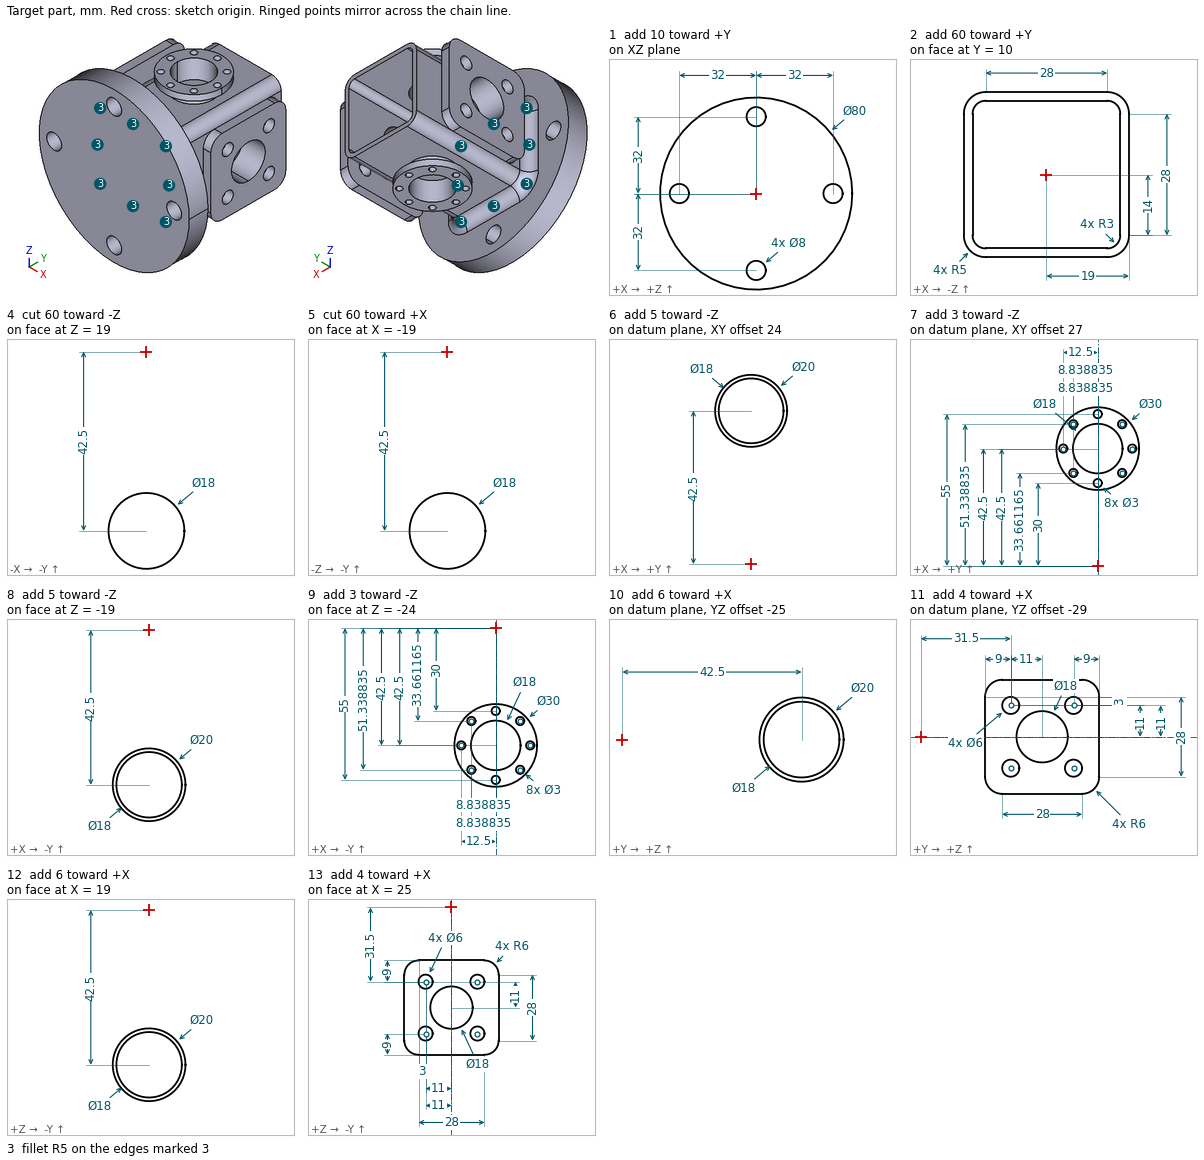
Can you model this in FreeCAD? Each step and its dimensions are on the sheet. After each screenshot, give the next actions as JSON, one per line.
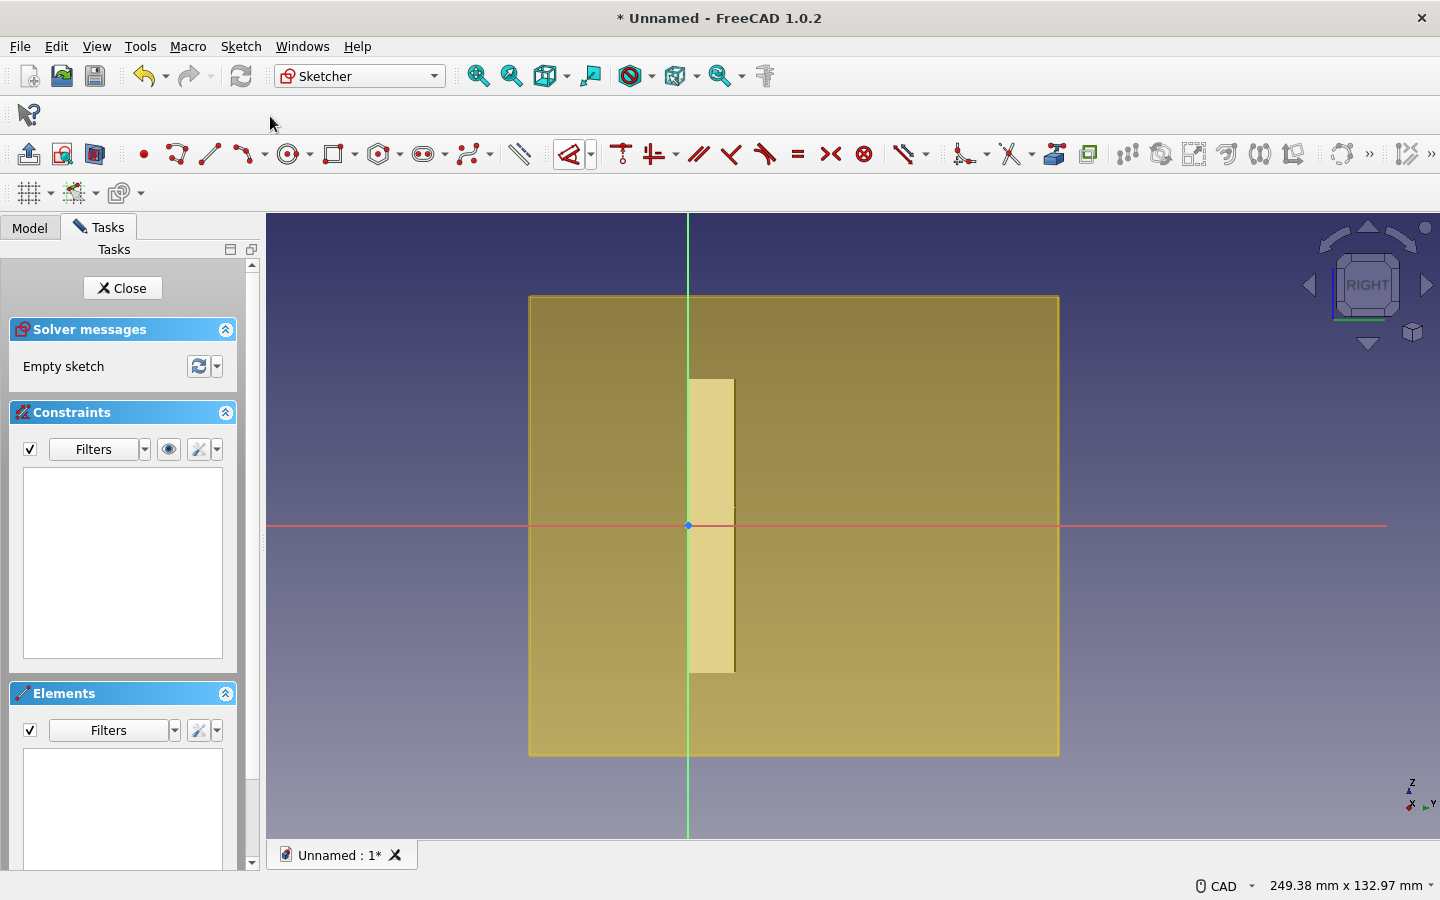
{"action": "scroll", "coordinate": [922, 526], "scroll_direction": "up", "scroll_amount": 7}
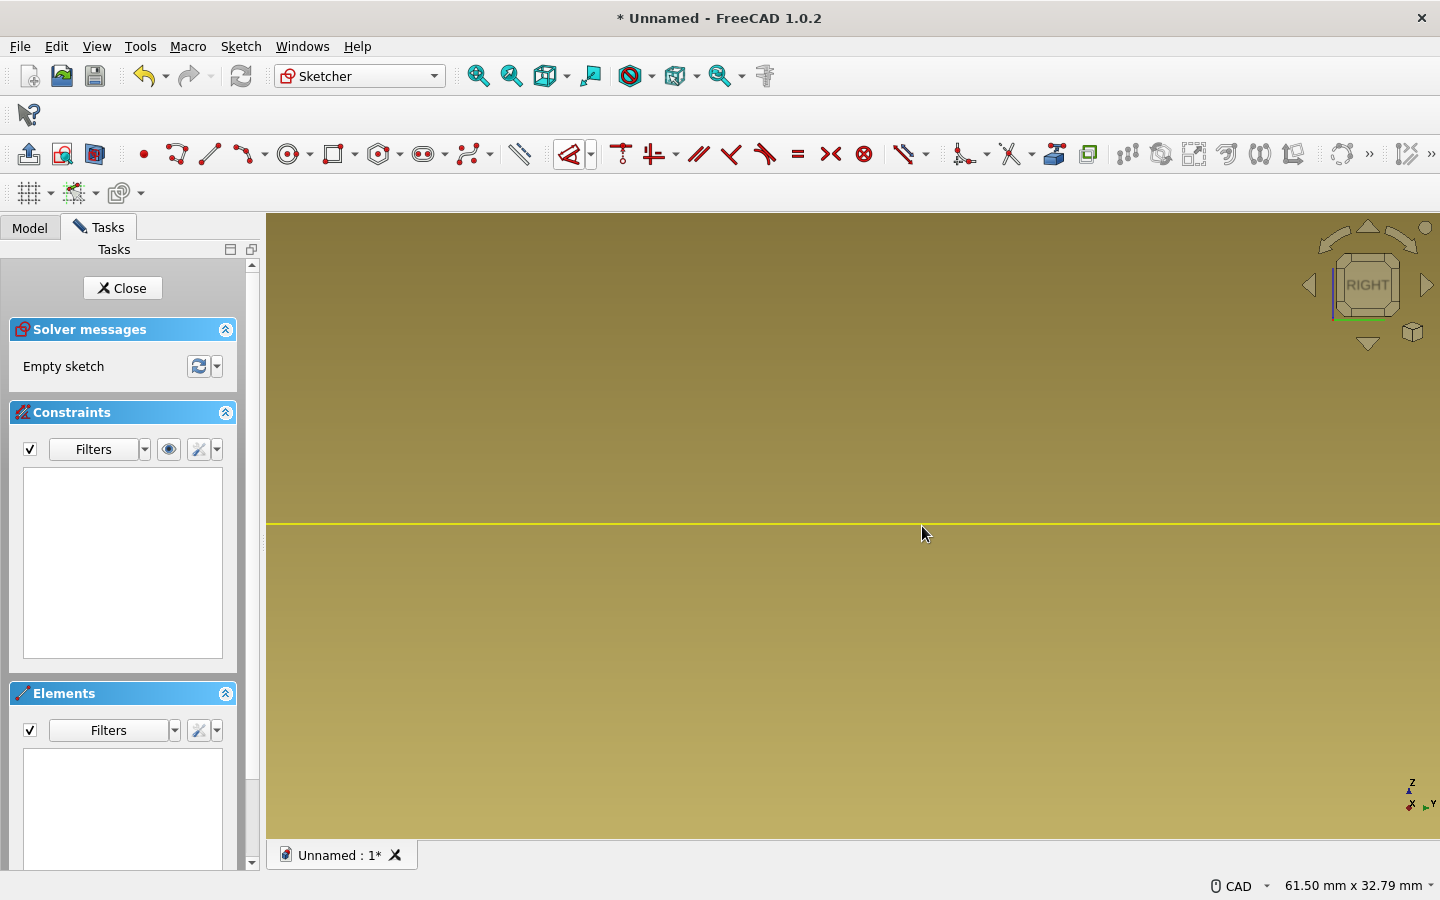
{"action": "key", "text": "g c"}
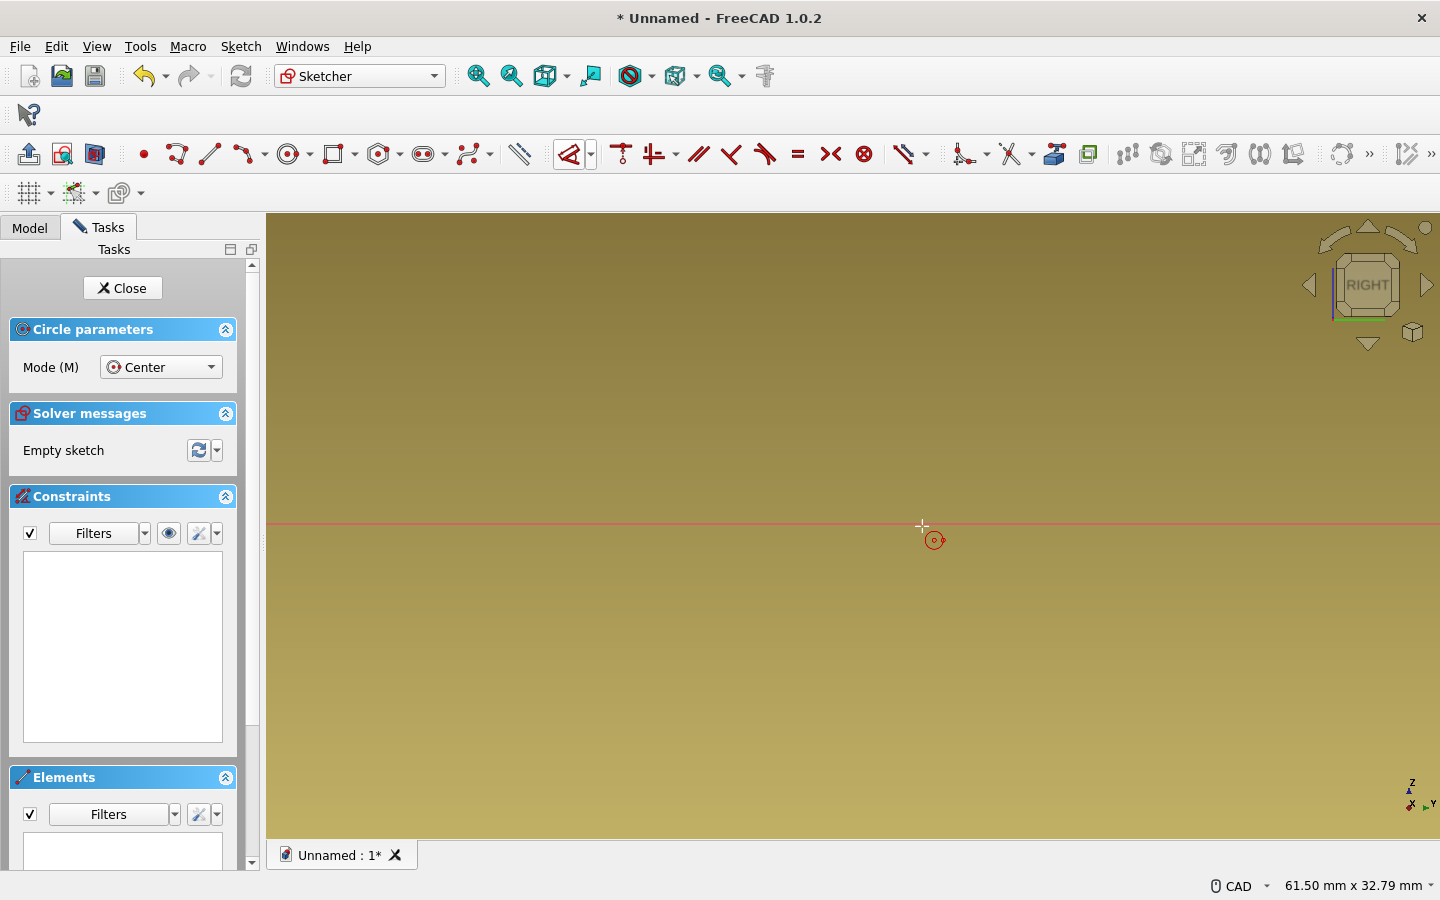
{"action": "left_click", "coordinate": [784, 524]}
{"action": "mouse_move", "coordinate": [919, 389]}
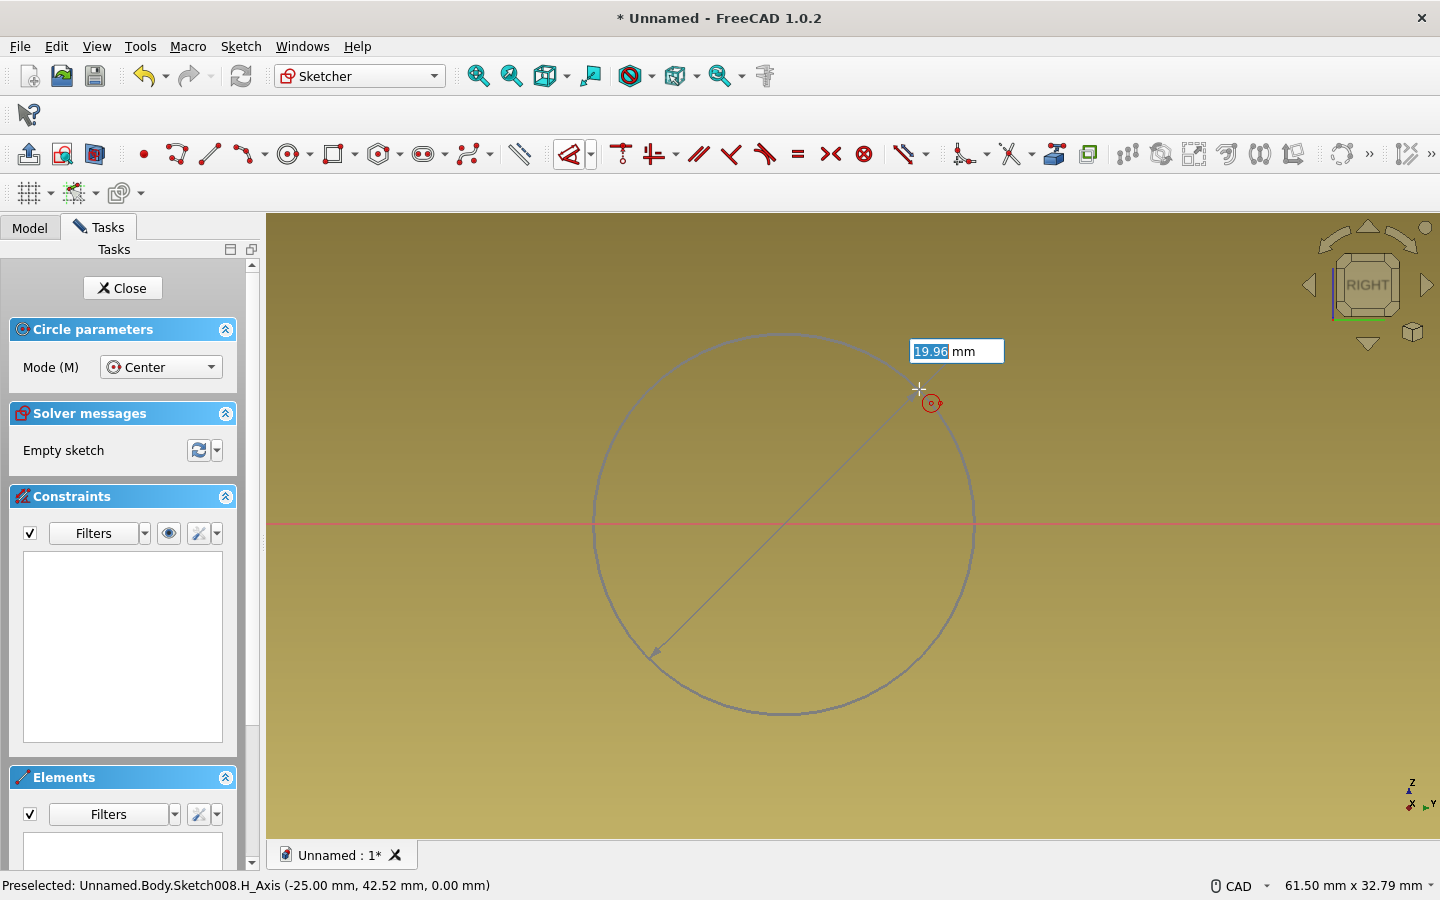
{"action": "type", "text": "20"}
{"action": "key", "text": "Return"}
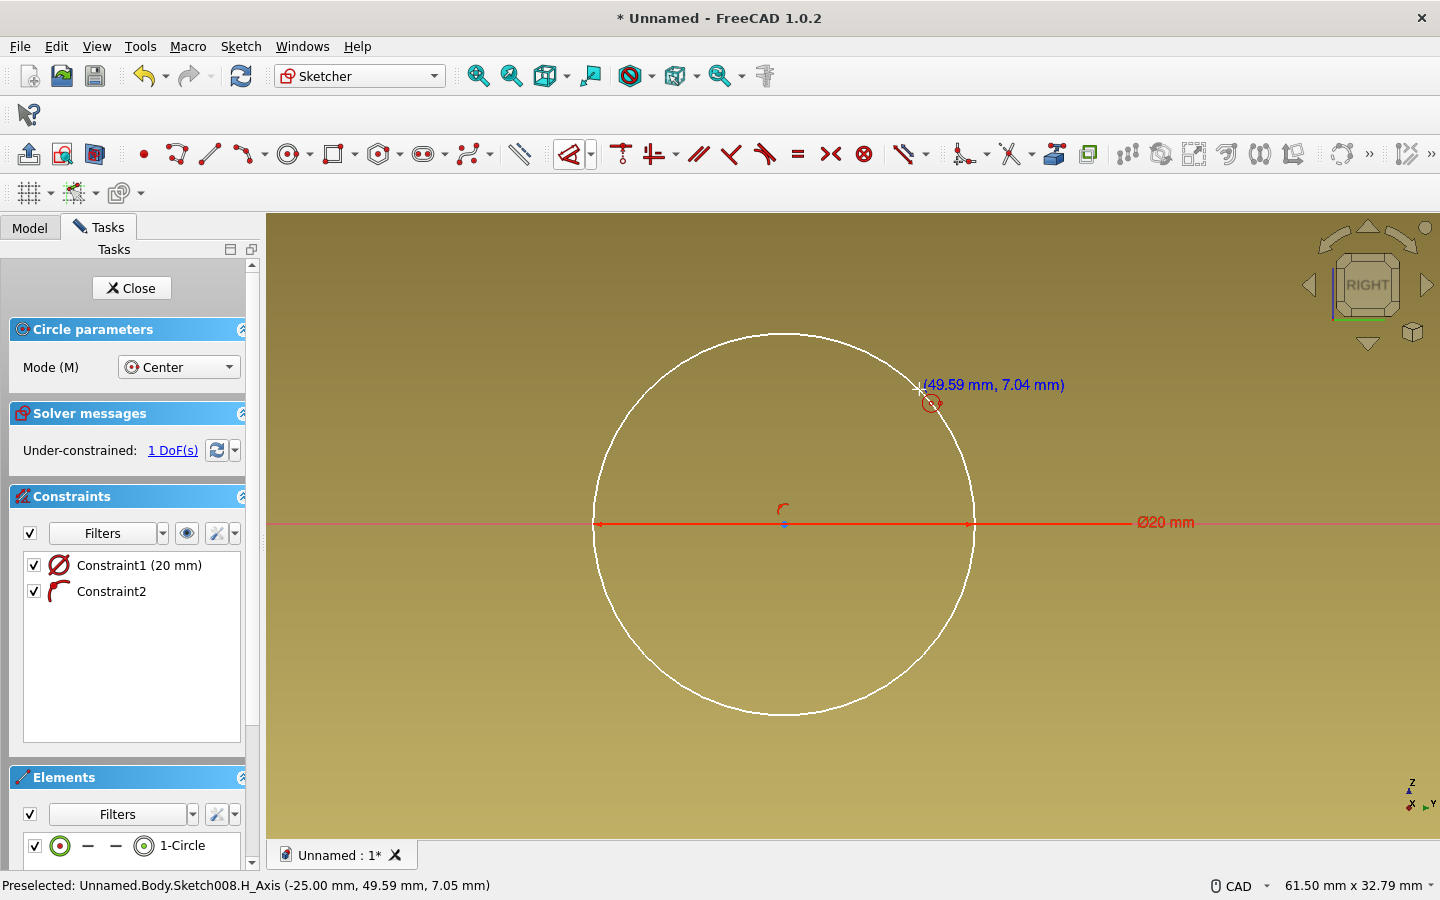
{"action": "left_click", "coordinate": [784, 524]}
{"action": "mouse_move", "coordinate": [905, 403]}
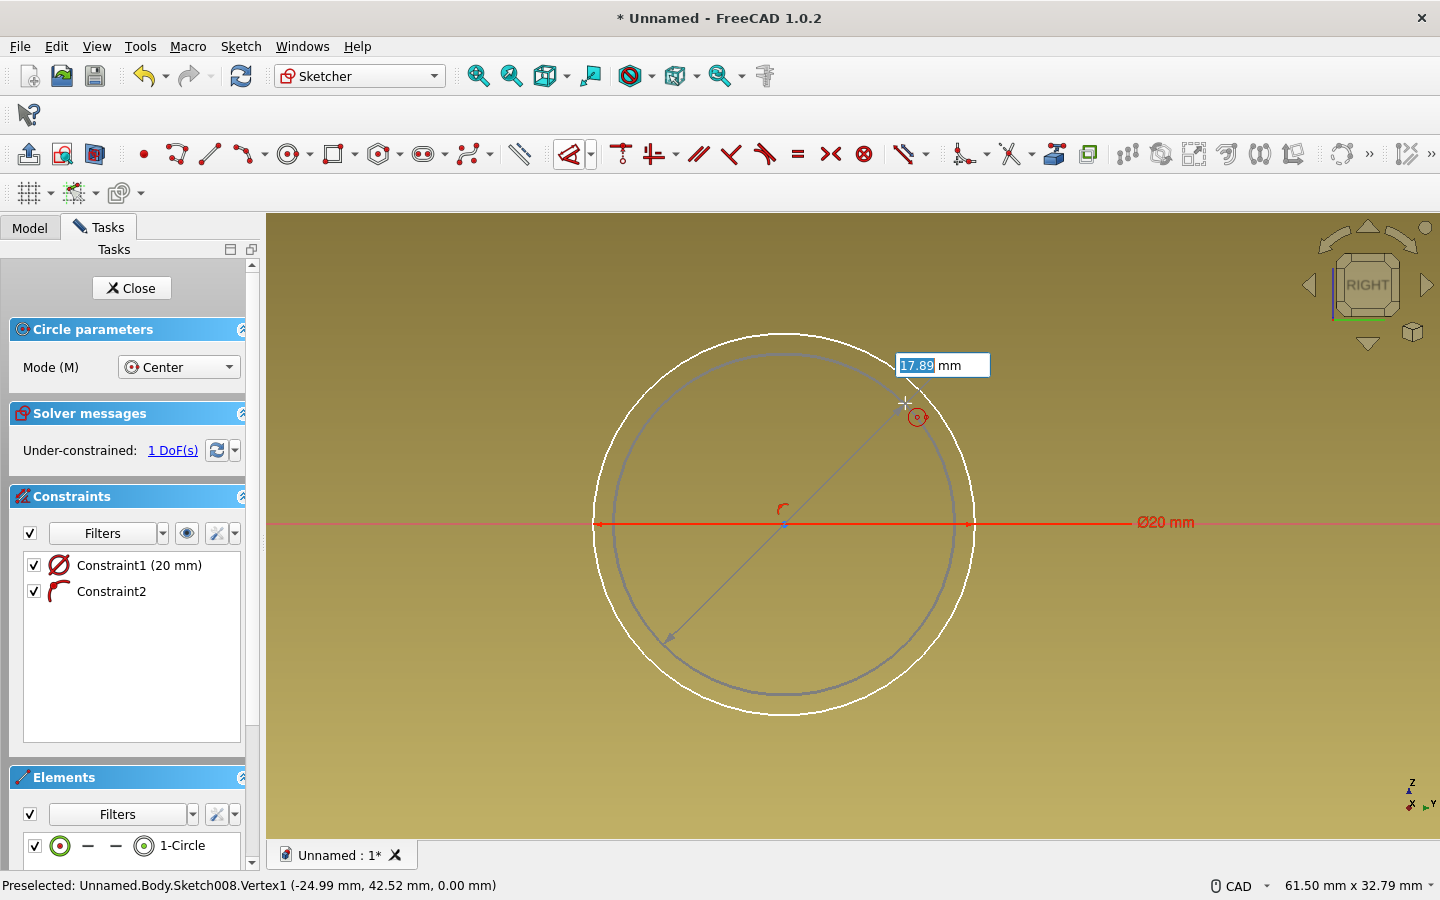
{"action": "type", "text": "18"}
{"action": "key", "text": "Return"}
{"action": "key", "text": "Escape"}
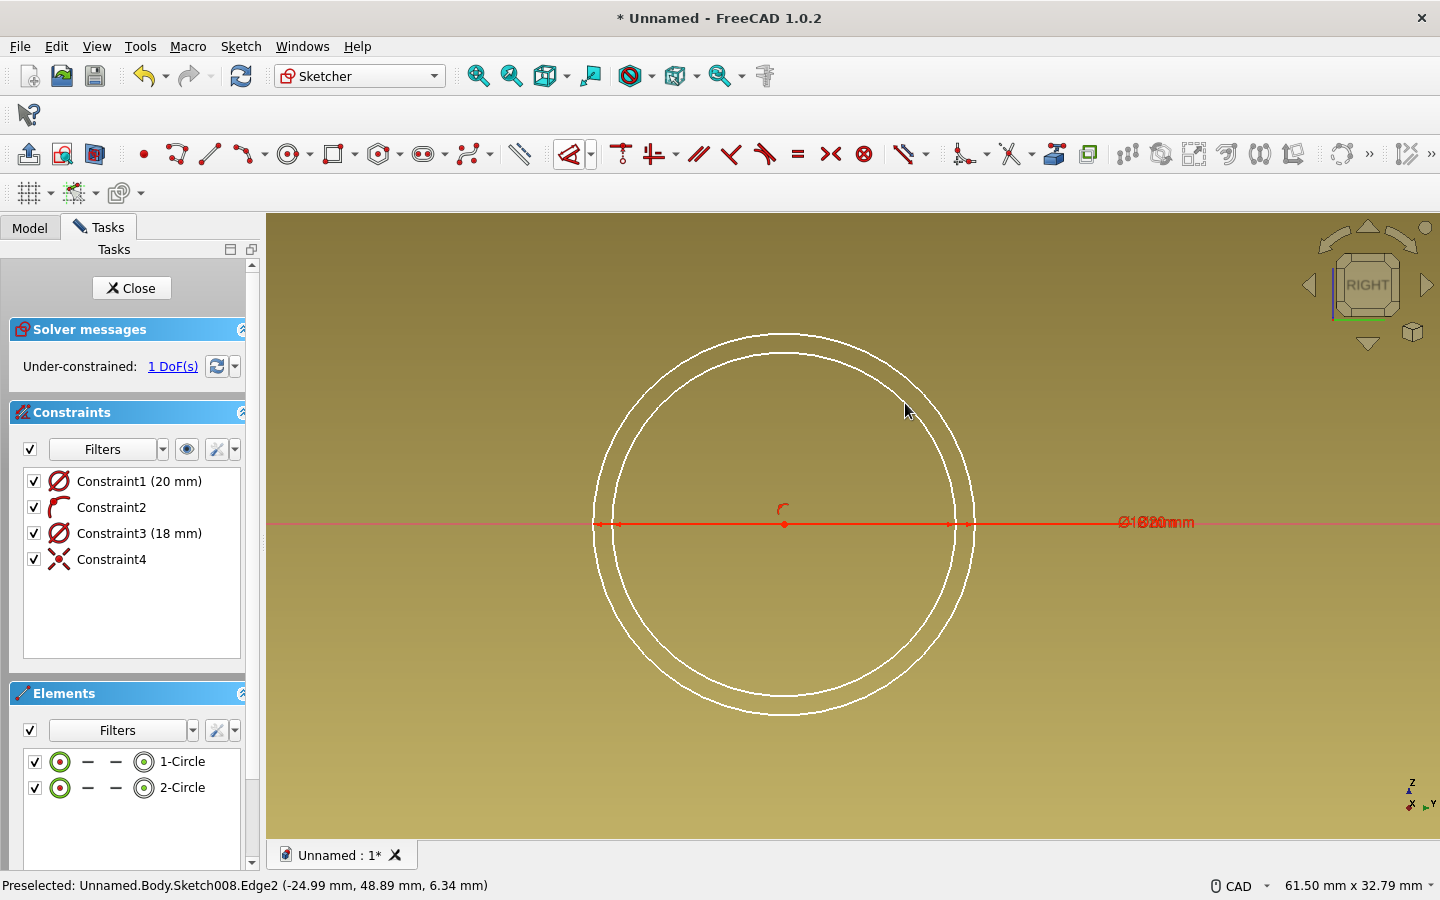
{"action": "left_click", "coordinate": [784, 524]}